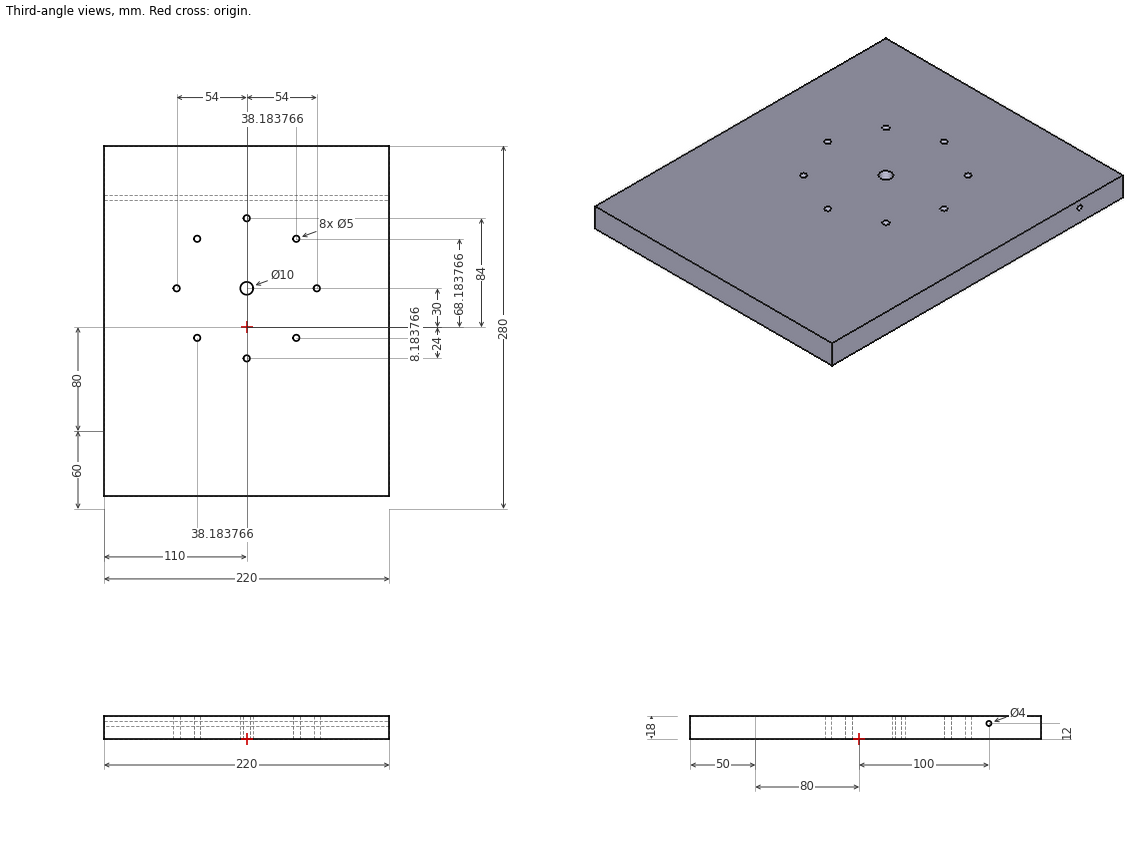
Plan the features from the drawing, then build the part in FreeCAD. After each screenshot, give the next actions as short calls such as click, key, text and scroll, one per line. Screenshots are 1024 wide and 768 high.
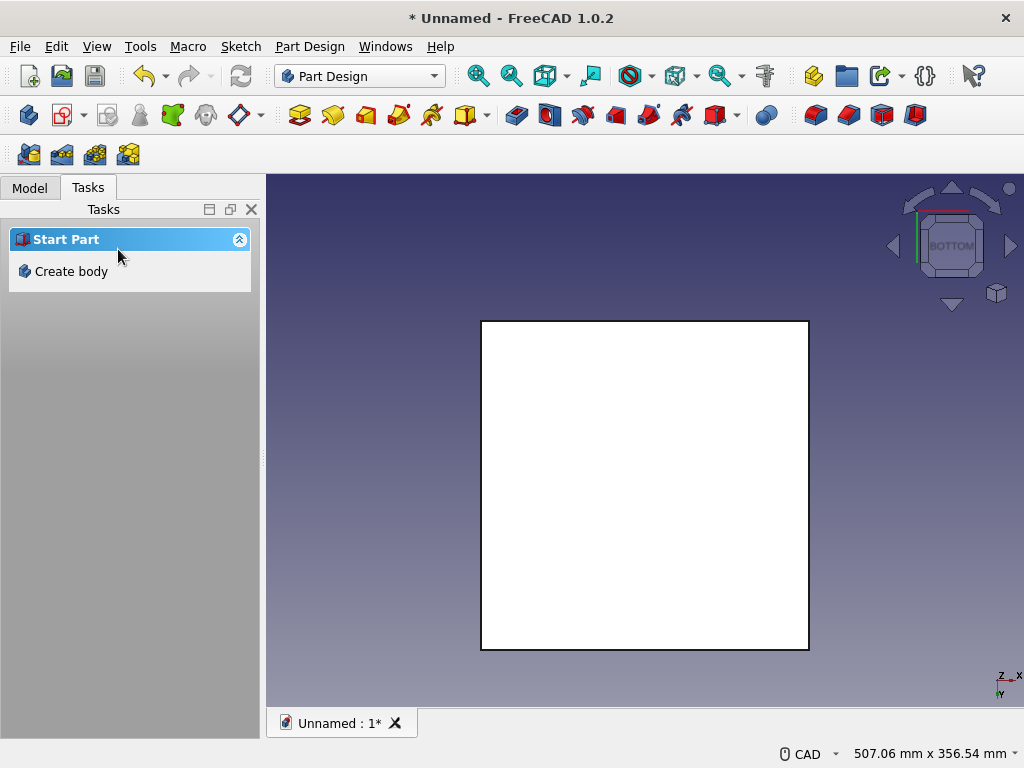
click(645, 484)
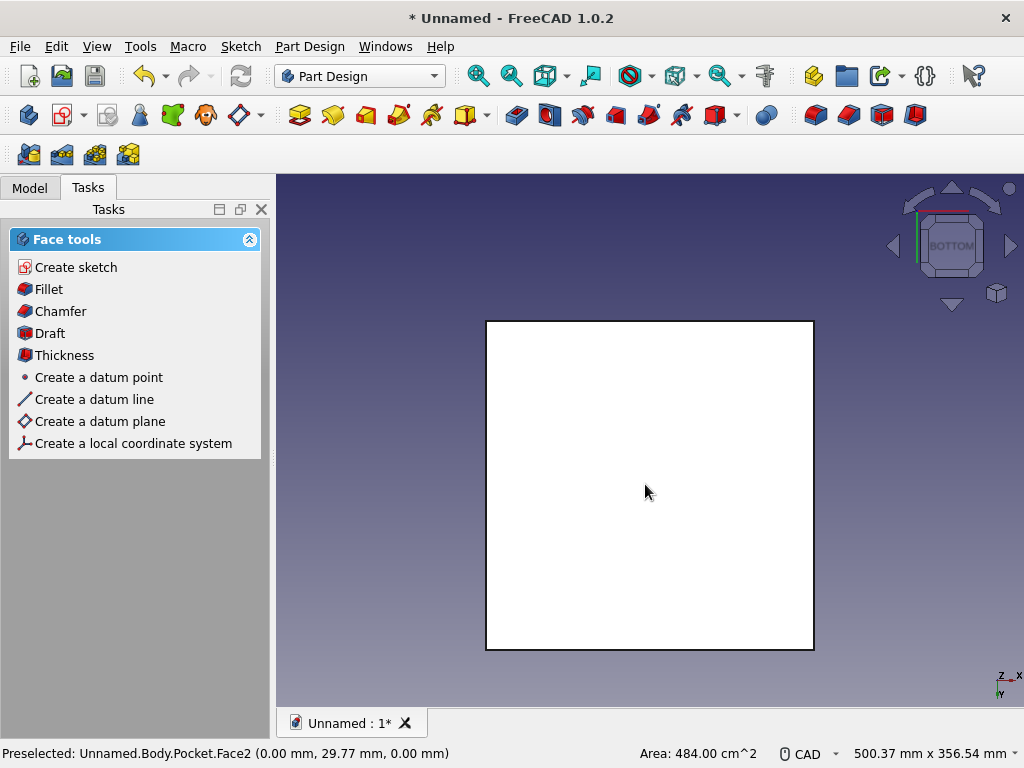
click(62, 116)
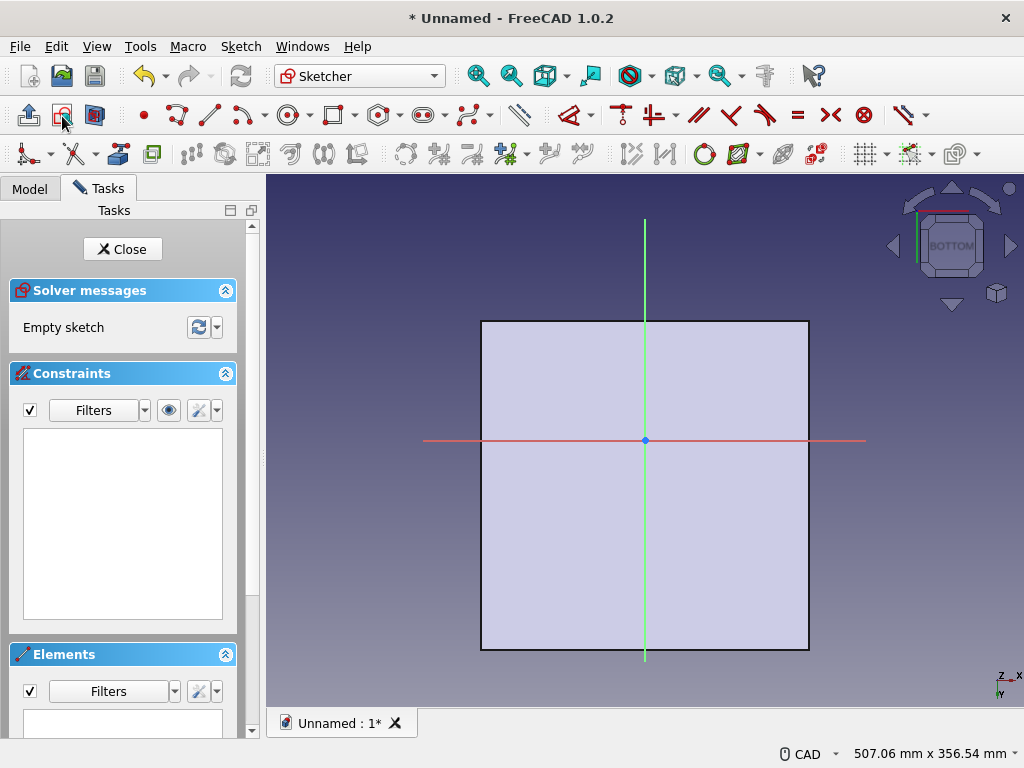
scroll(649, 488, up, 15)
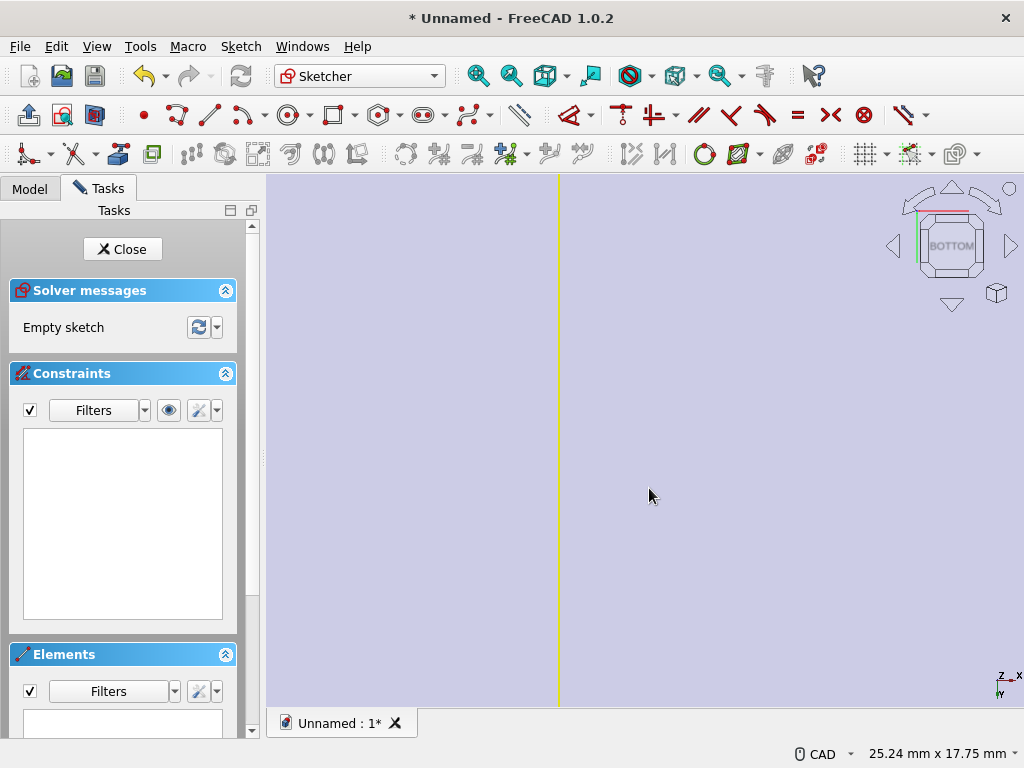
key(g)
key(c)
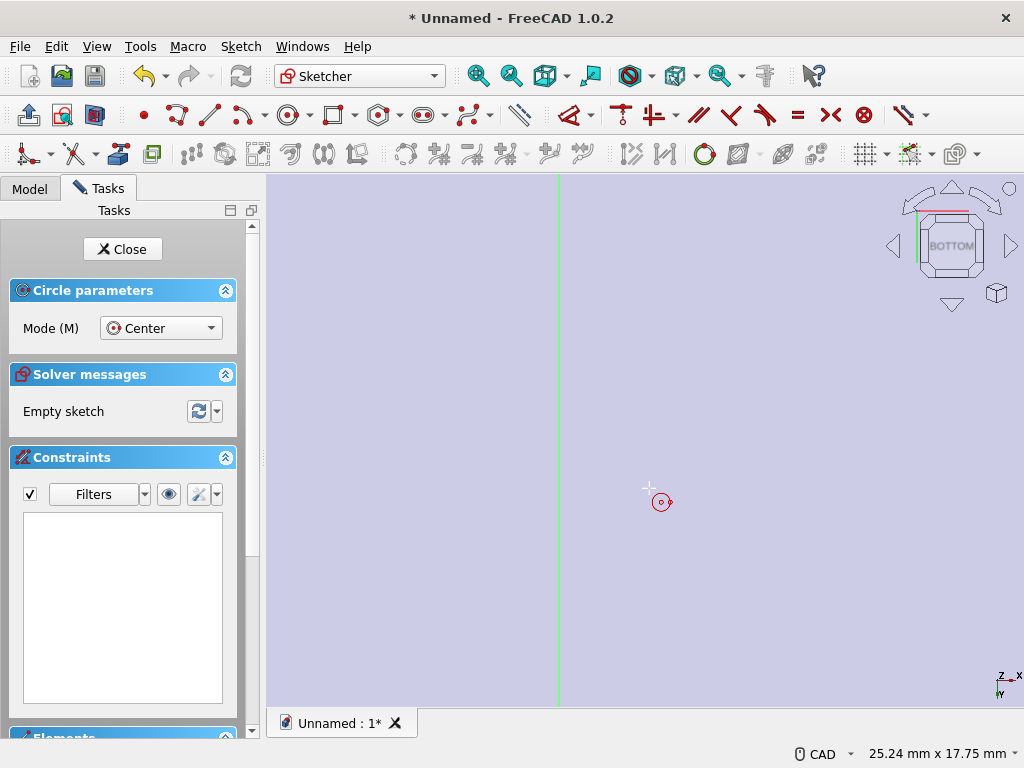
click(559, 423)
click(665, 317)
key(Escape)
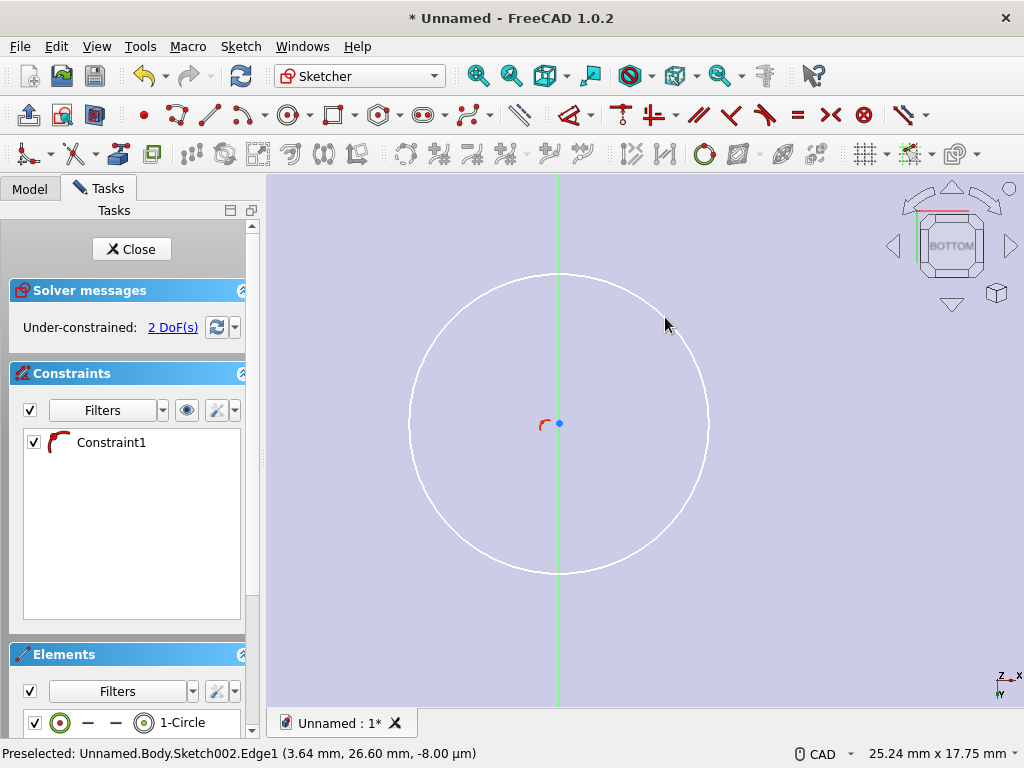
key(d)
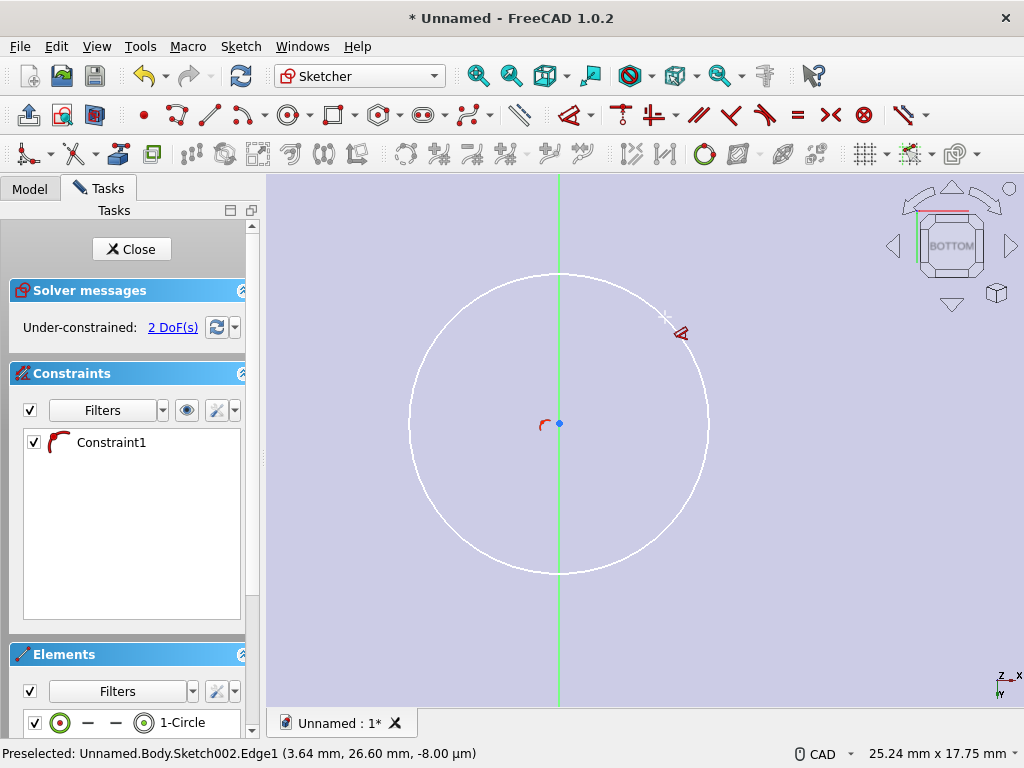
click(665, 318)
click(688, 295)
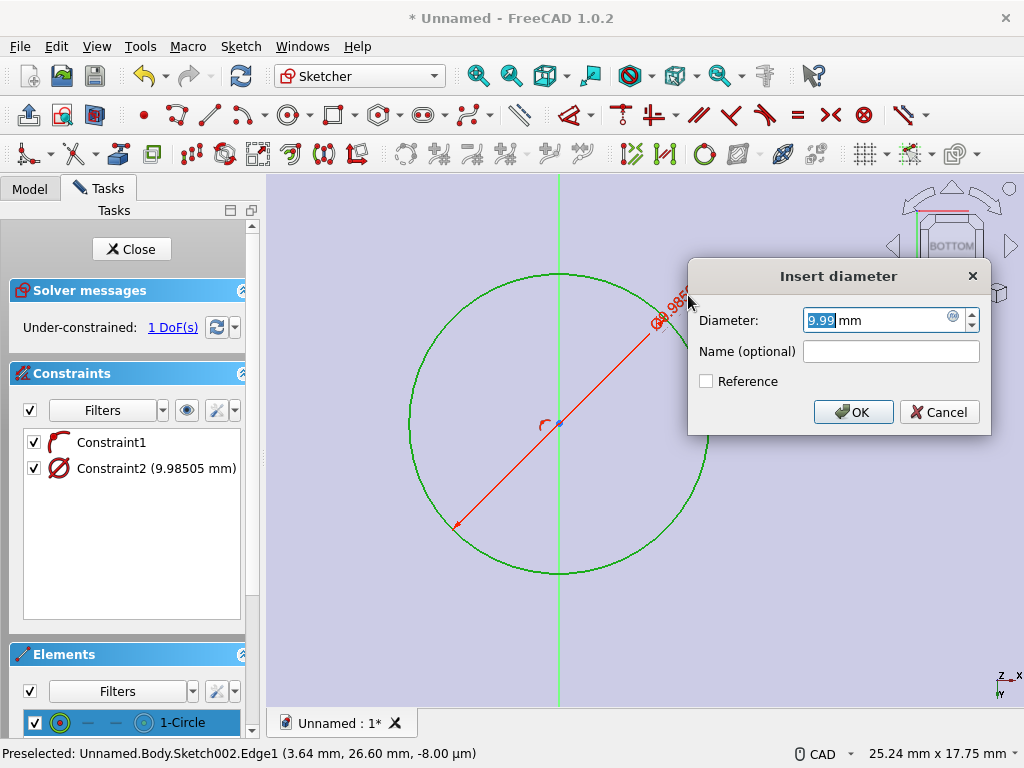
text(10)
key(Return)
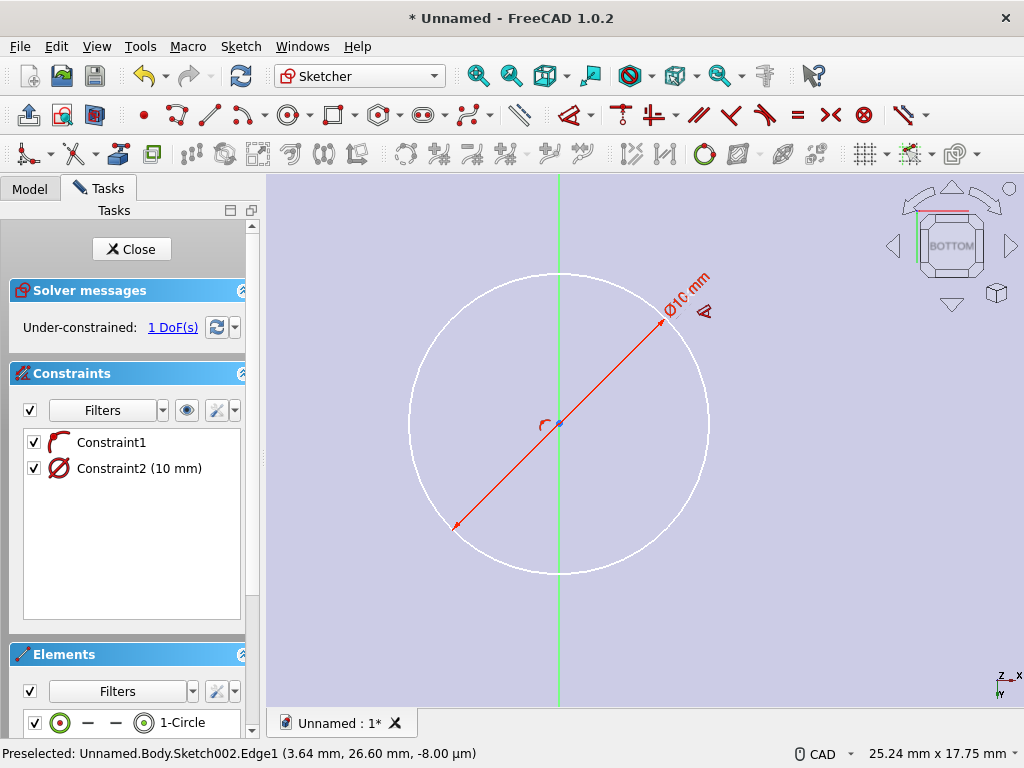
click(559, 424)
click(593, 313)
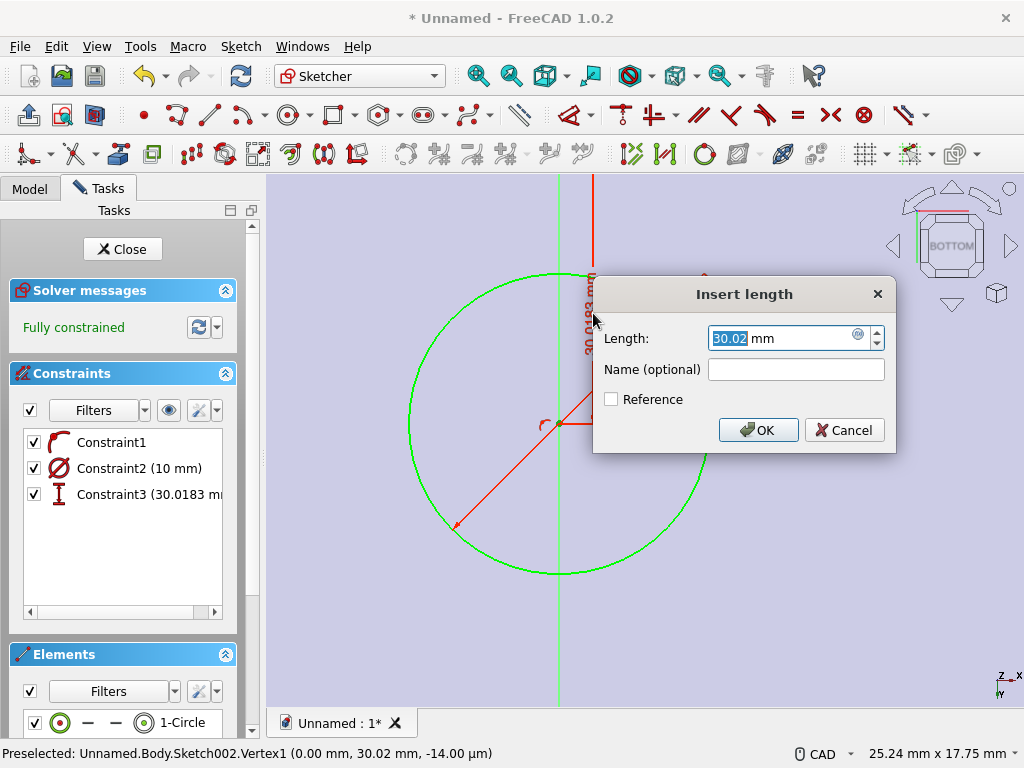
text(30)
key(Return)
key(Escape)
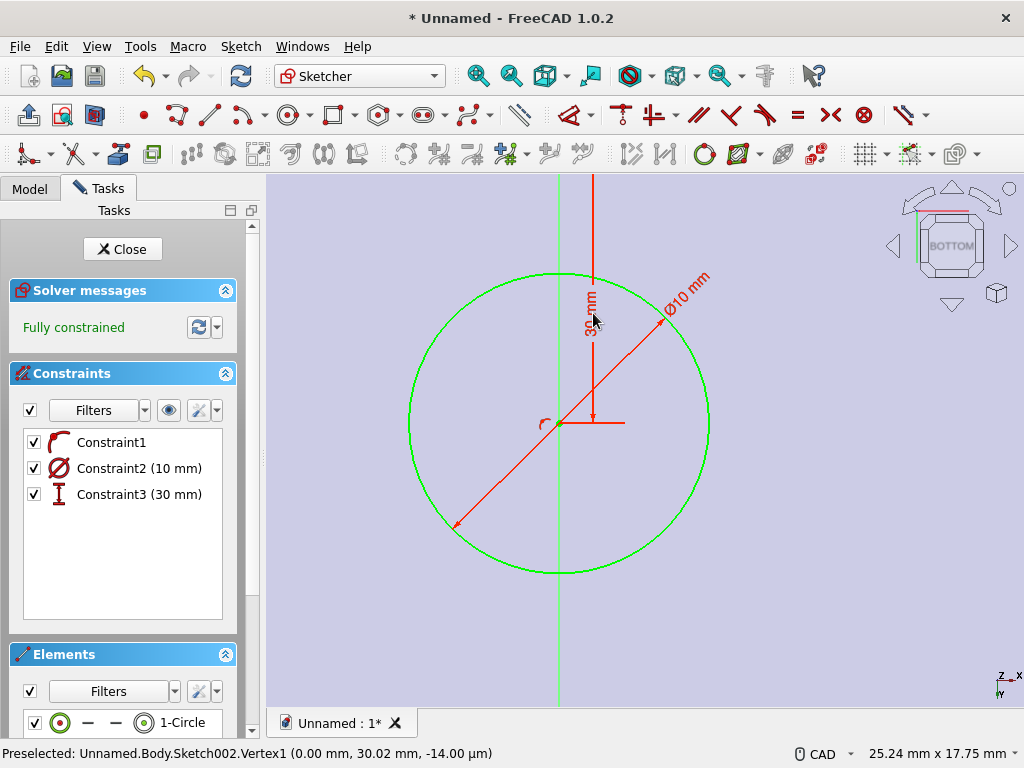
click(123, 249)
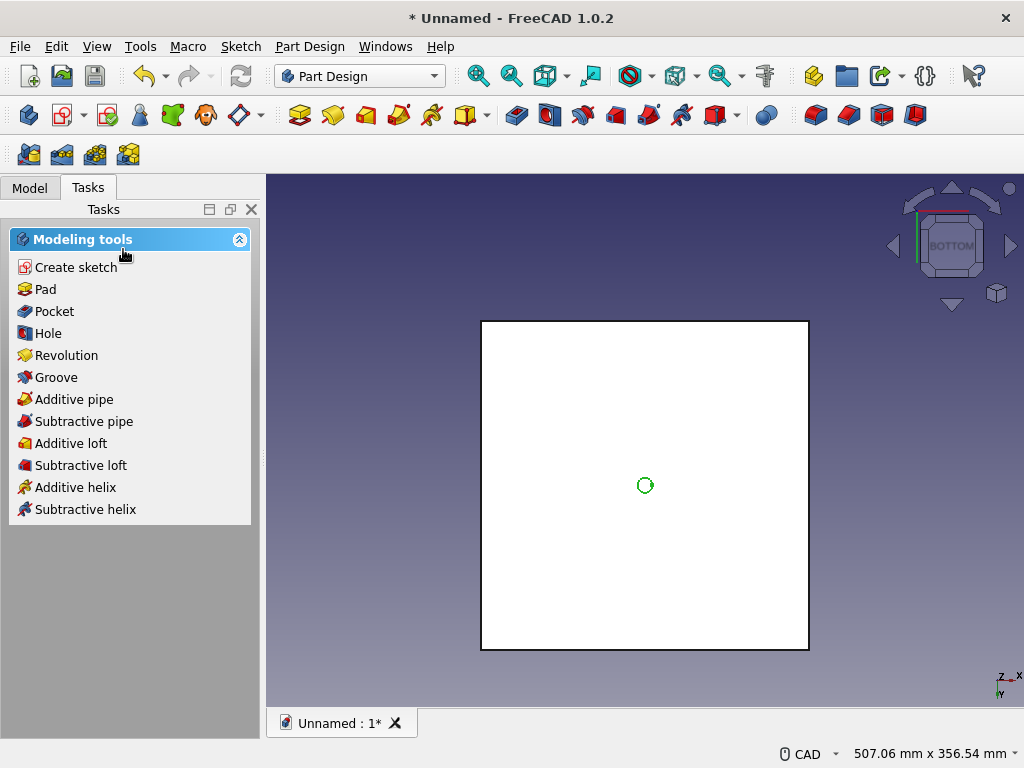
click(517, 116)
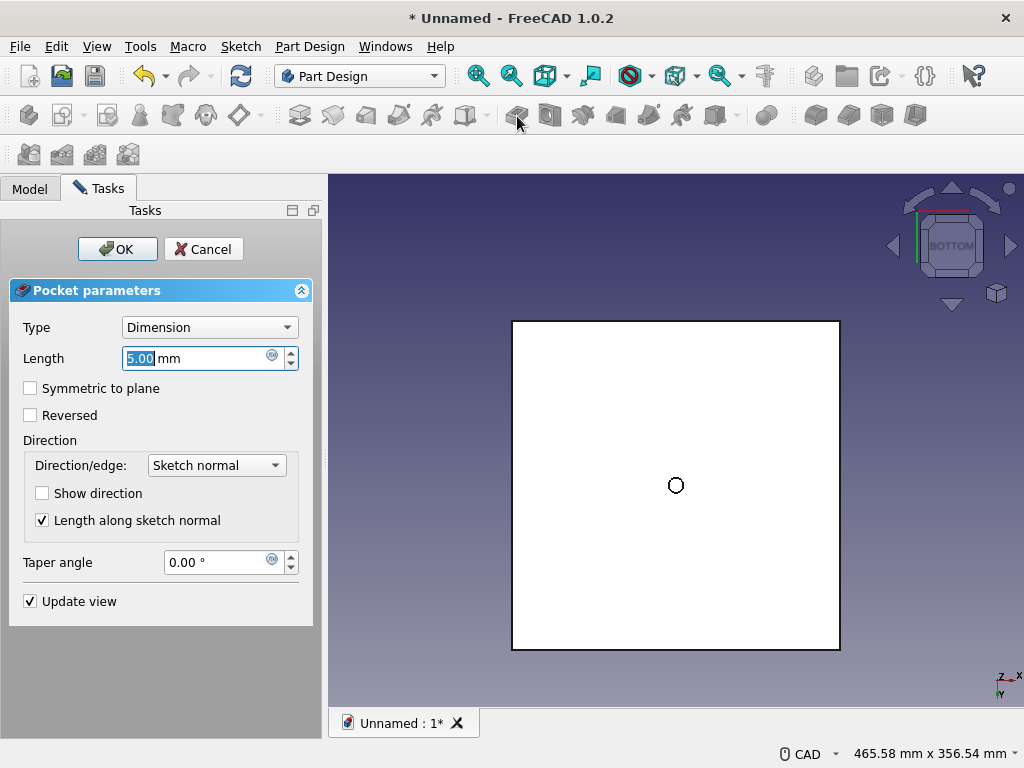
click(210, 328)